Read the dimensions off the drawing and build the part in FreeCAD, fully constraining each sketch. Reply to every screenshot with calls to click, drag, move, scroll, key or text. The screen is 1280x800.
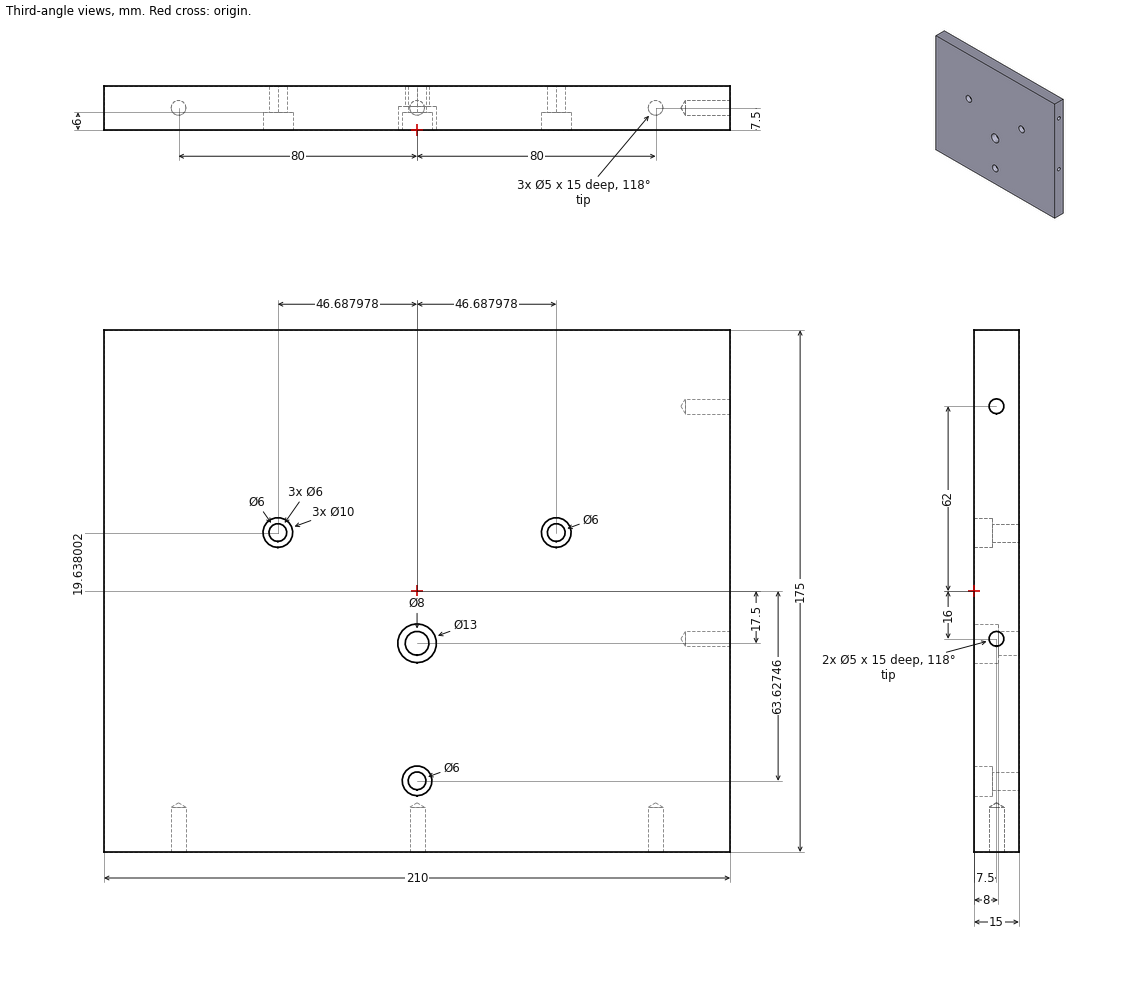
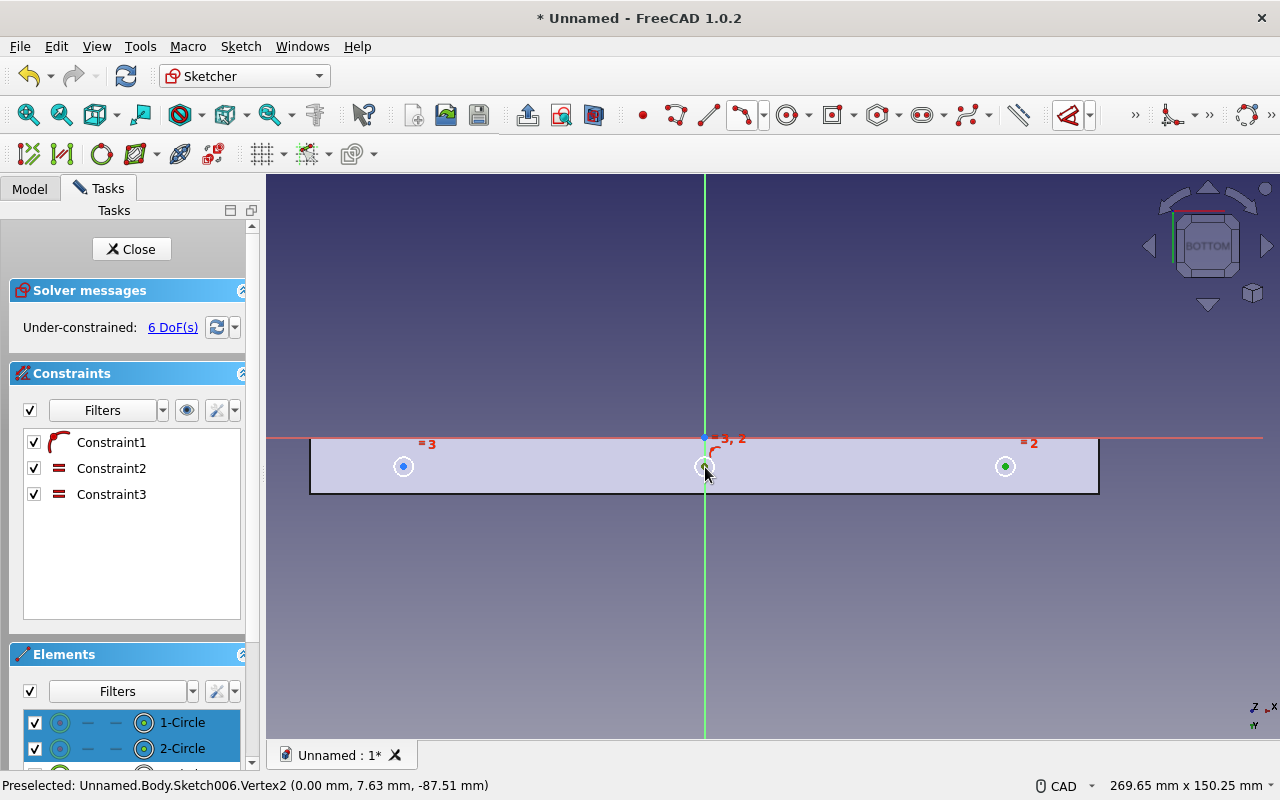
key(h)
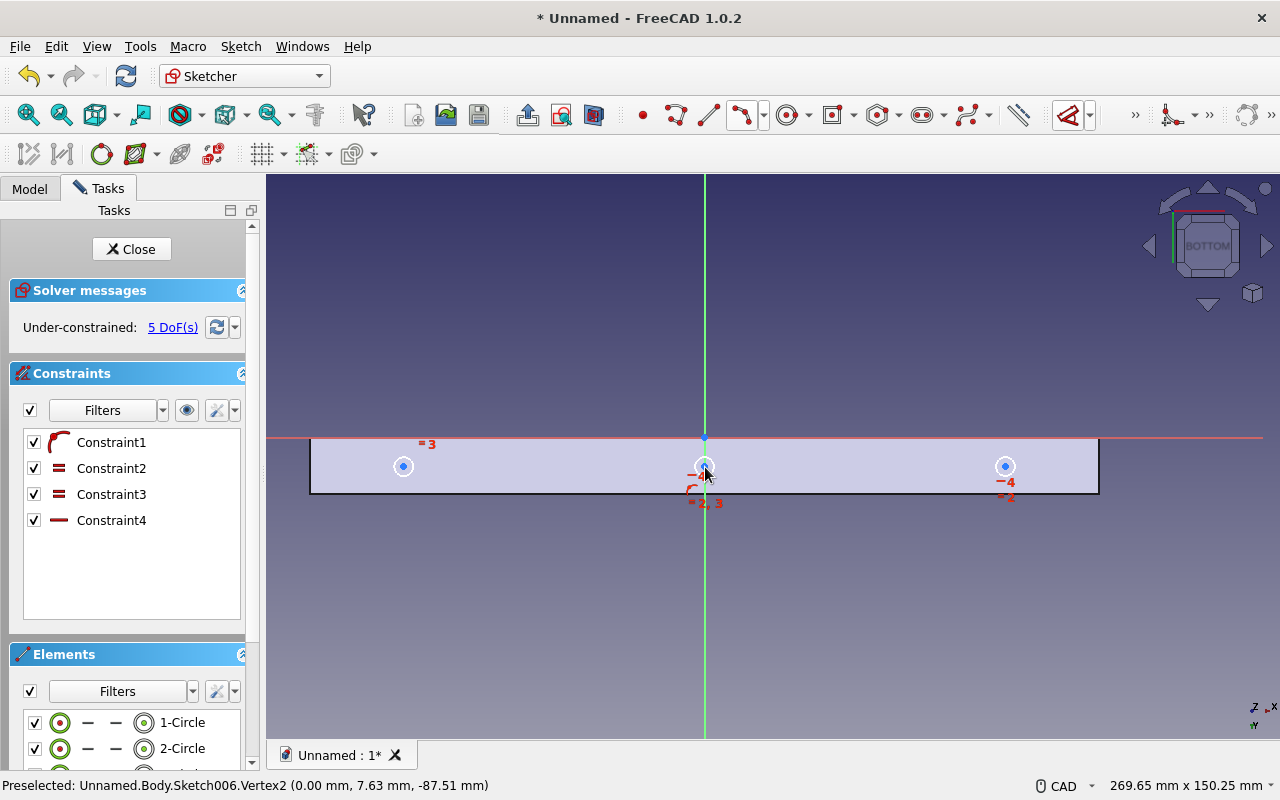
click(705, 467)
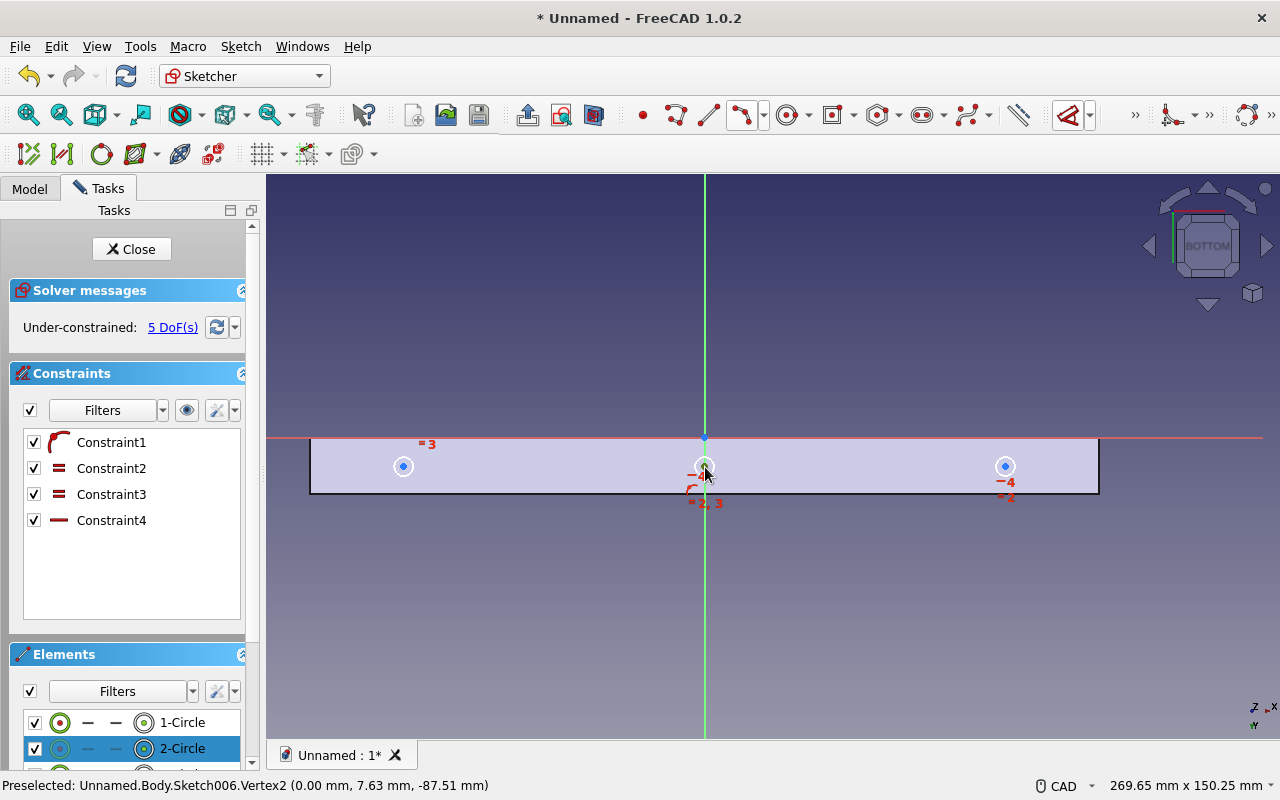
click(404, 467)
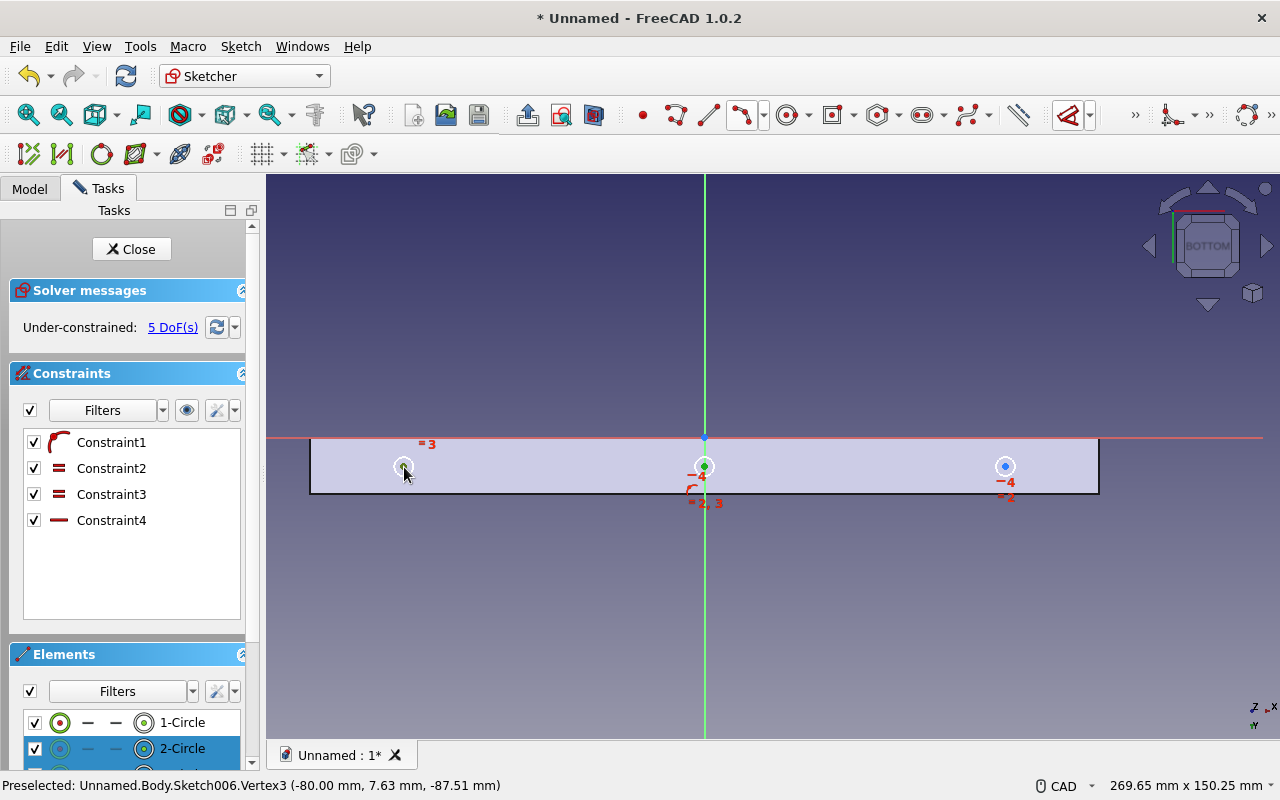
key(h)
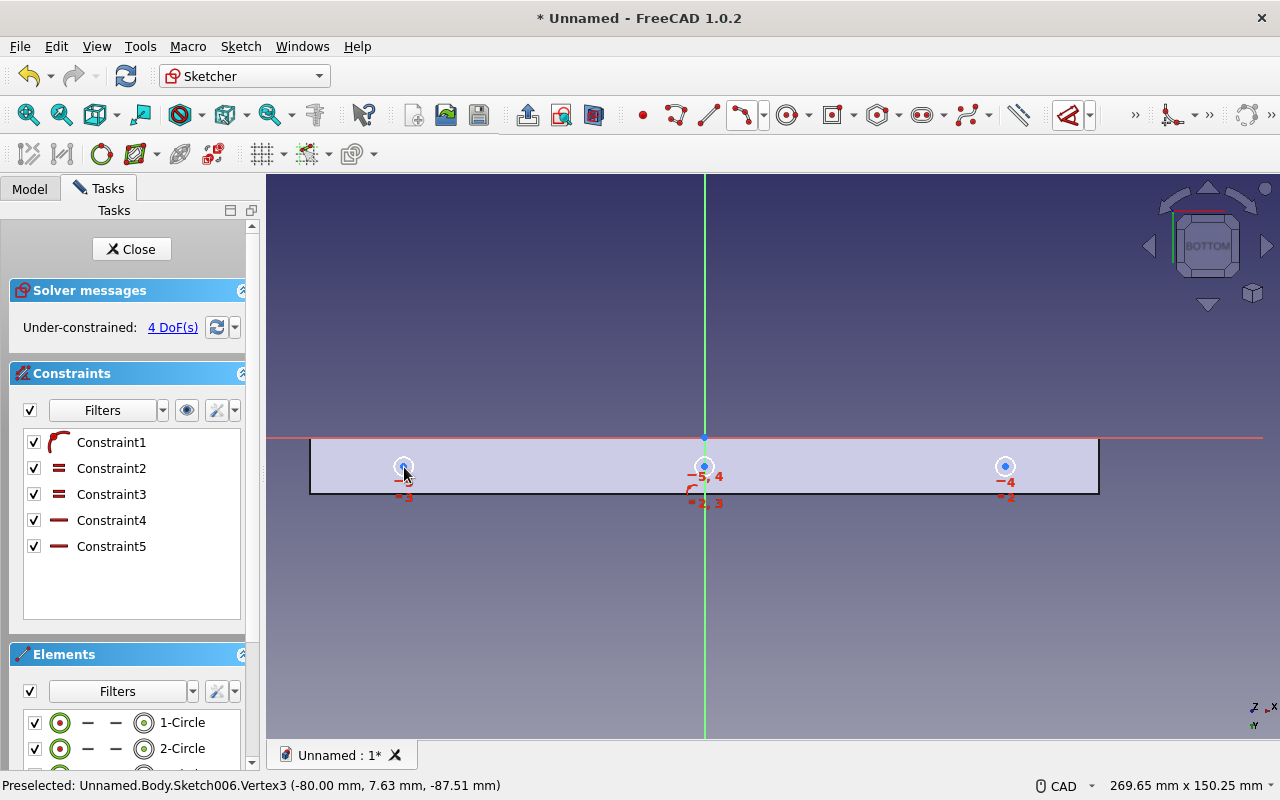
scroll(1012, 460, up, 4)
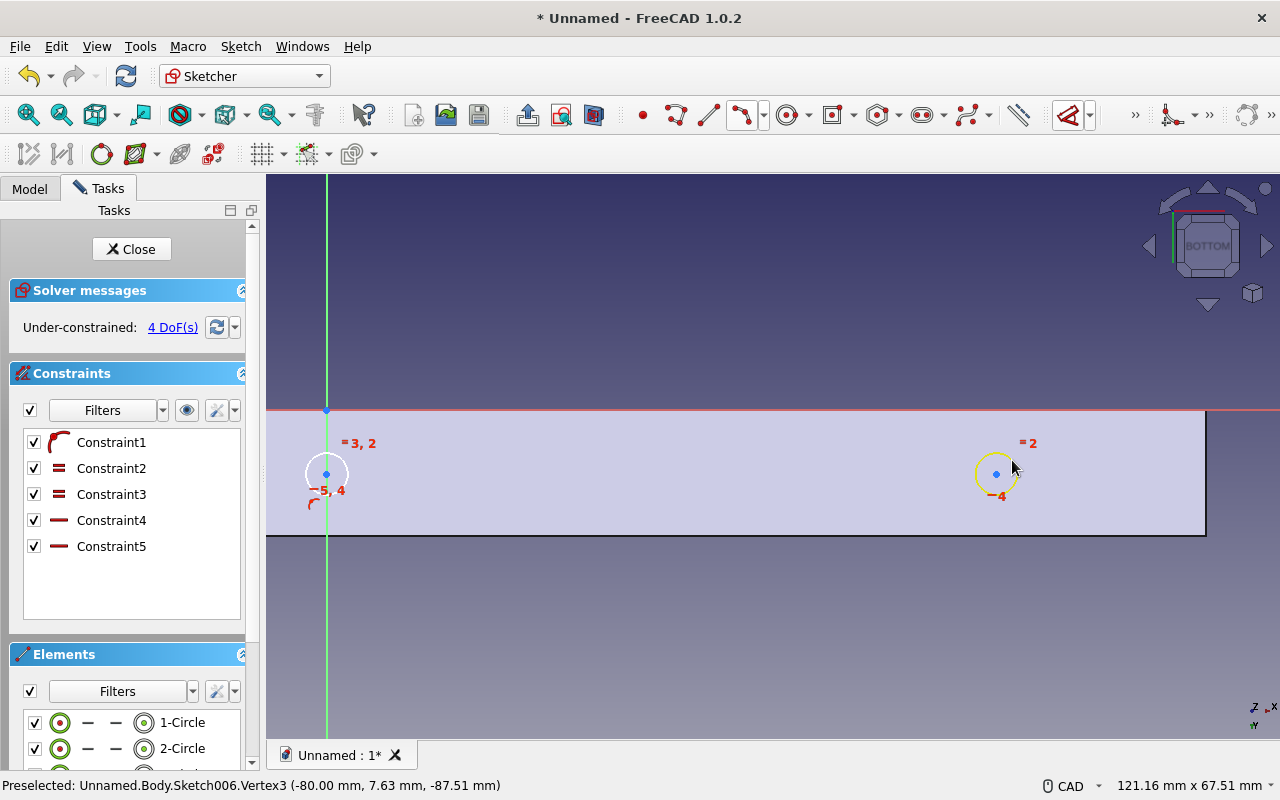
click(1011, 459)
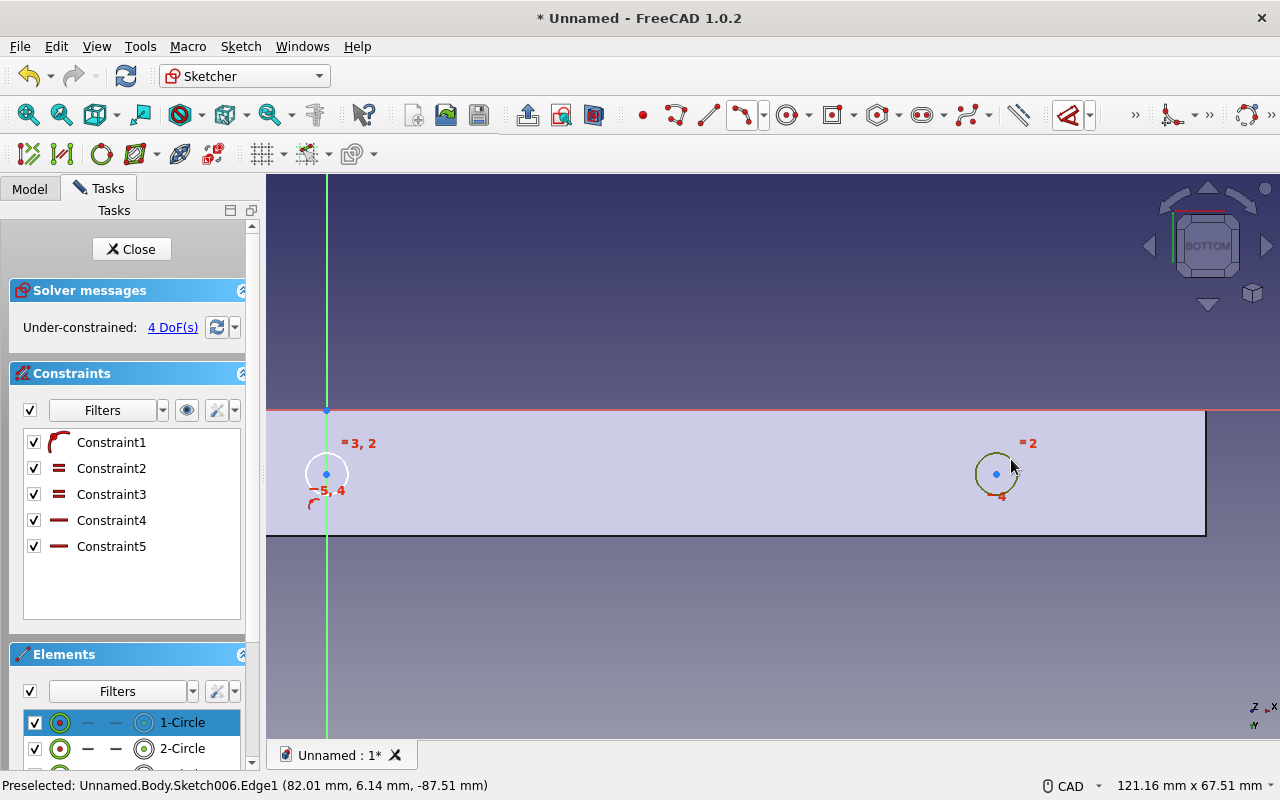
click(1090, 116)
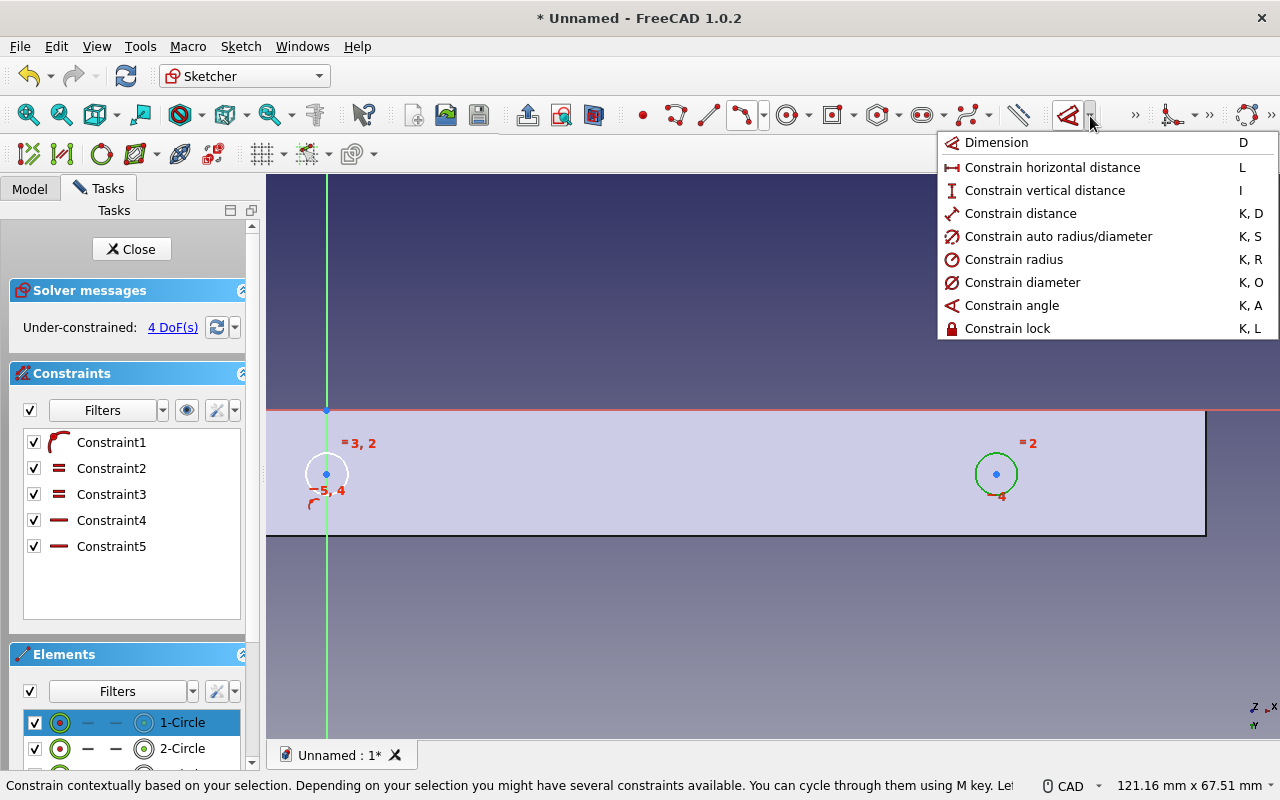
click(1108, 282)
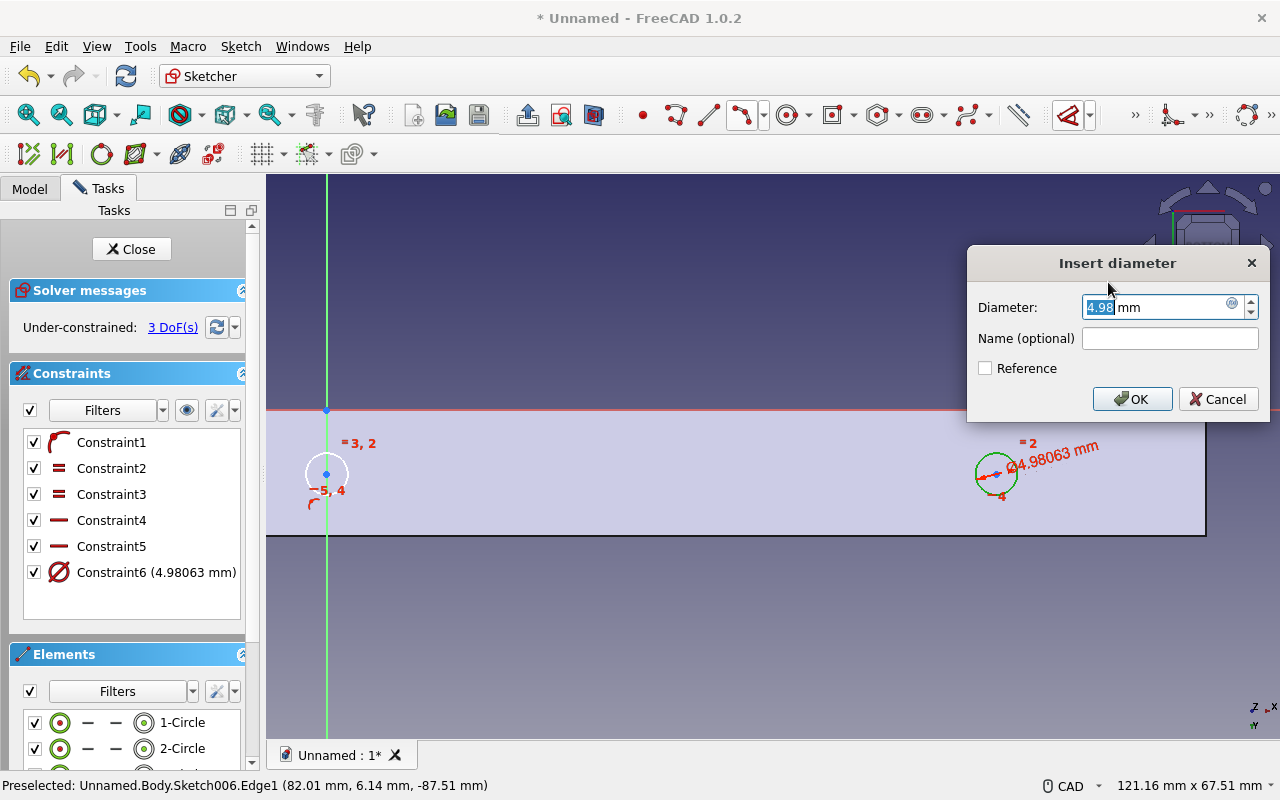
text(5)
key(Return)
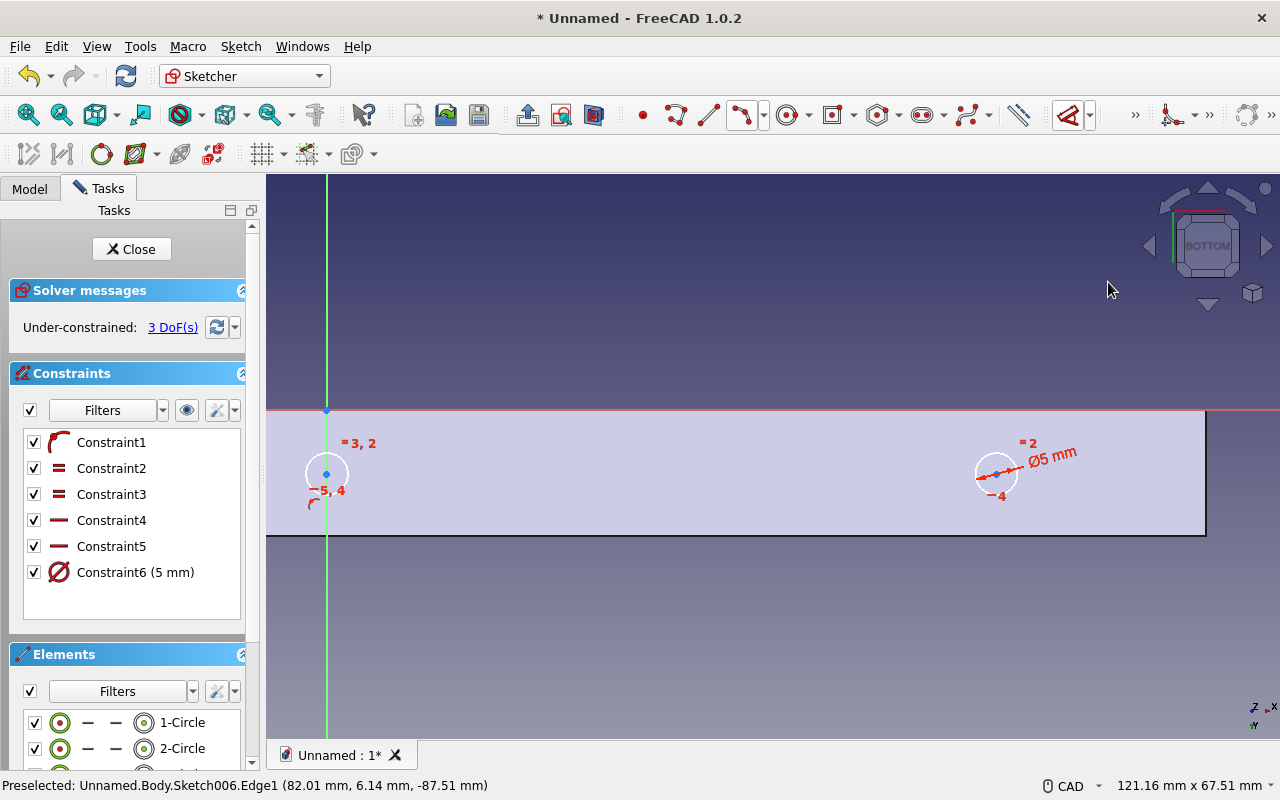
click(996, 474)